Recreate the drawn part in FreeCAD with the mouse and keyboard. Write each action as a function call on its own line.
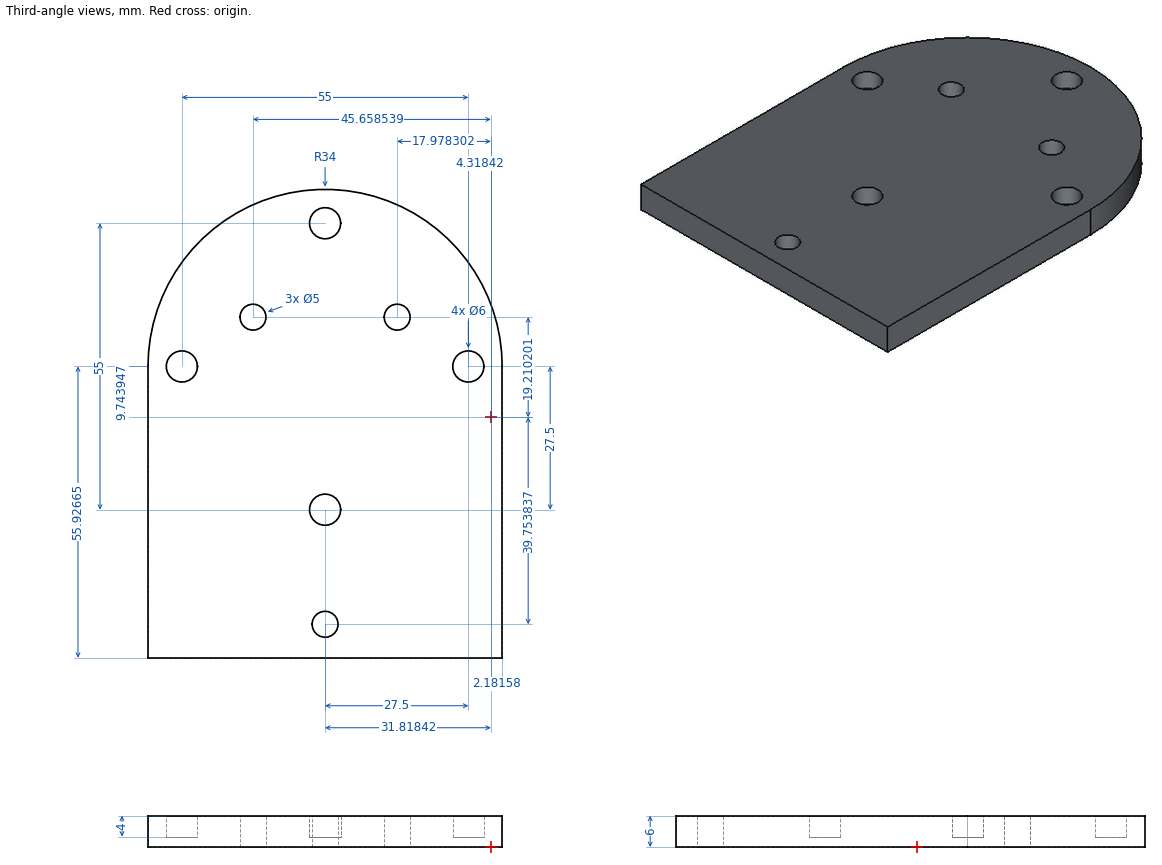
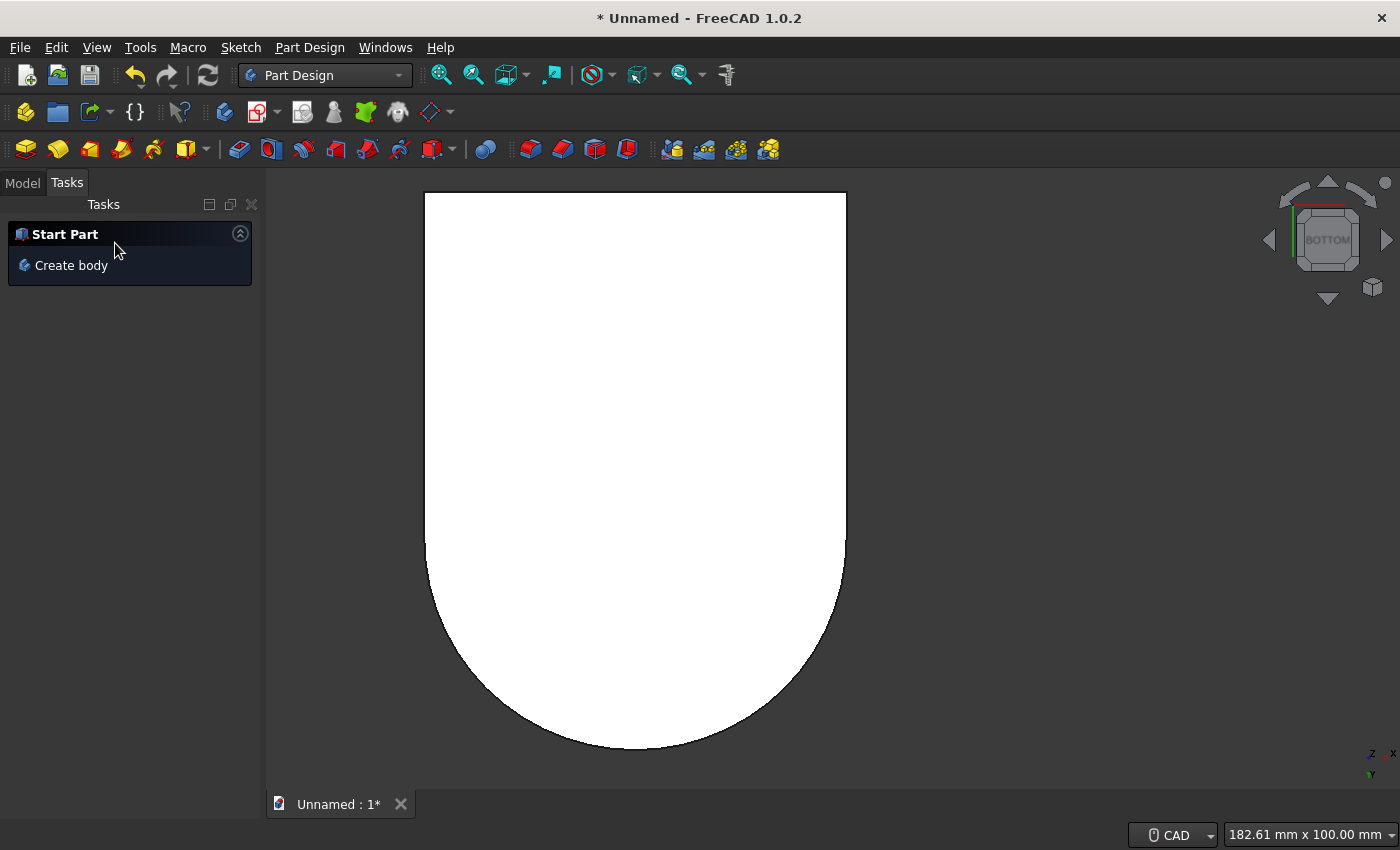
click(635, 470)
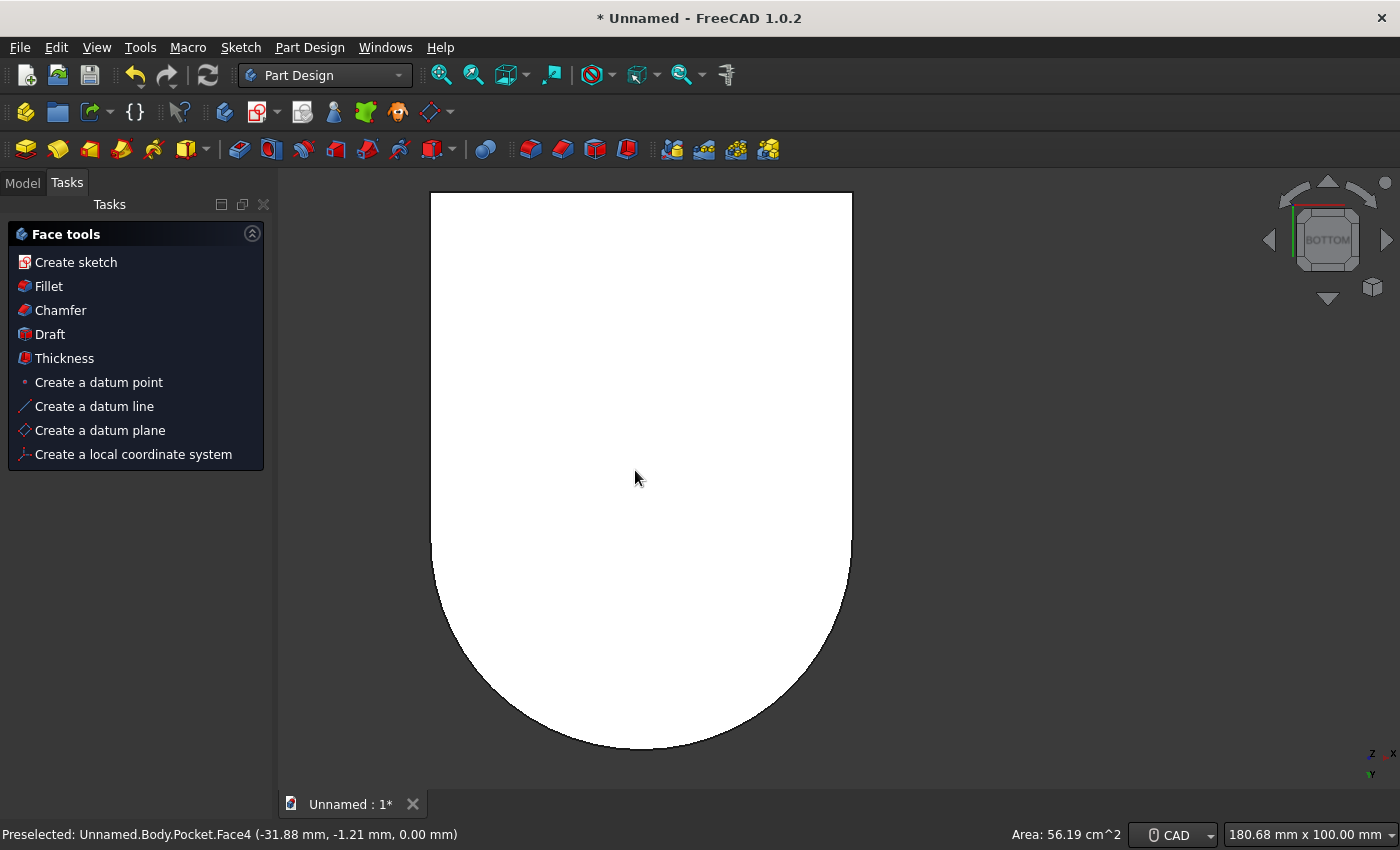
click(258, 112)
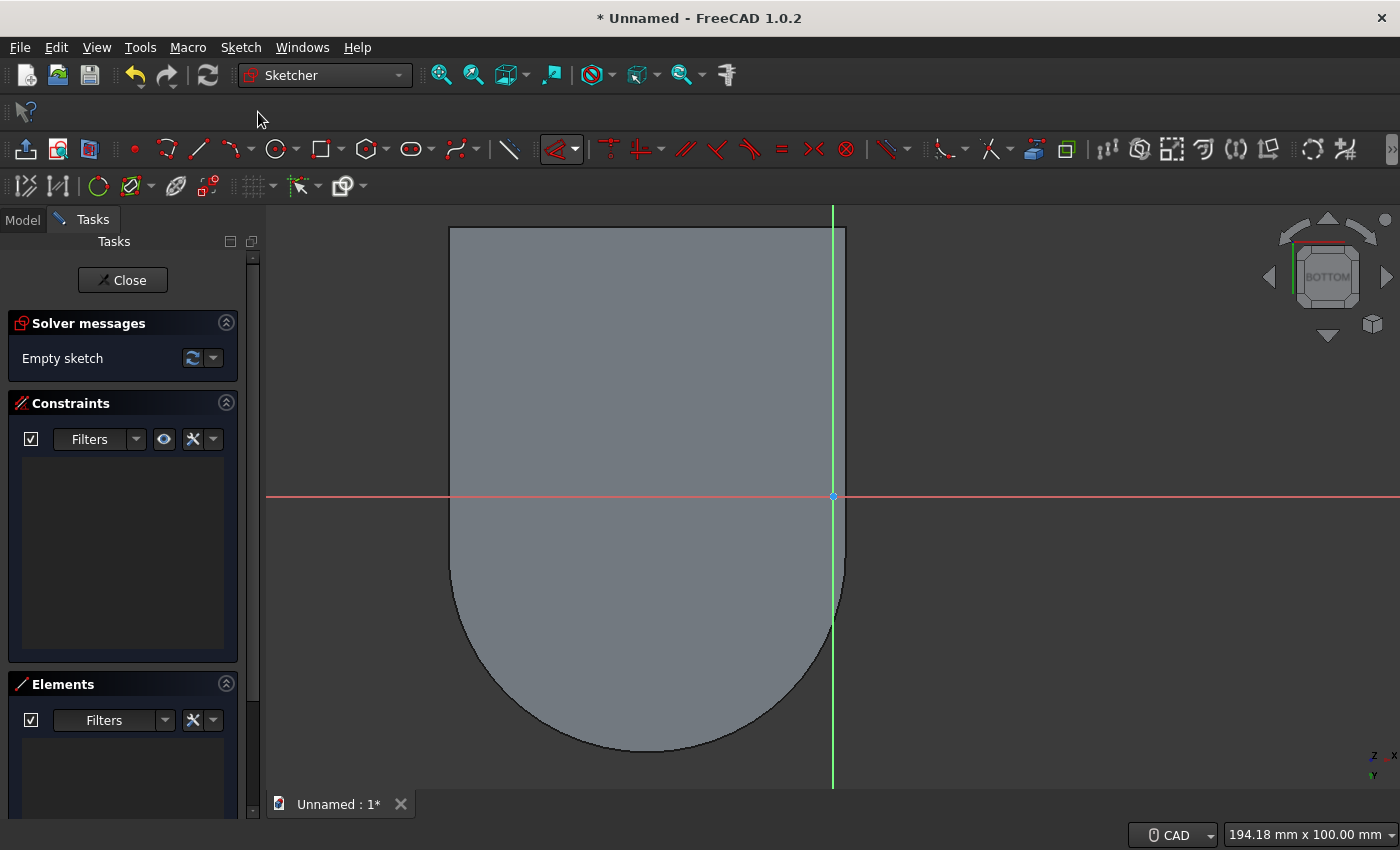
scroll(1090, 761, down, 1)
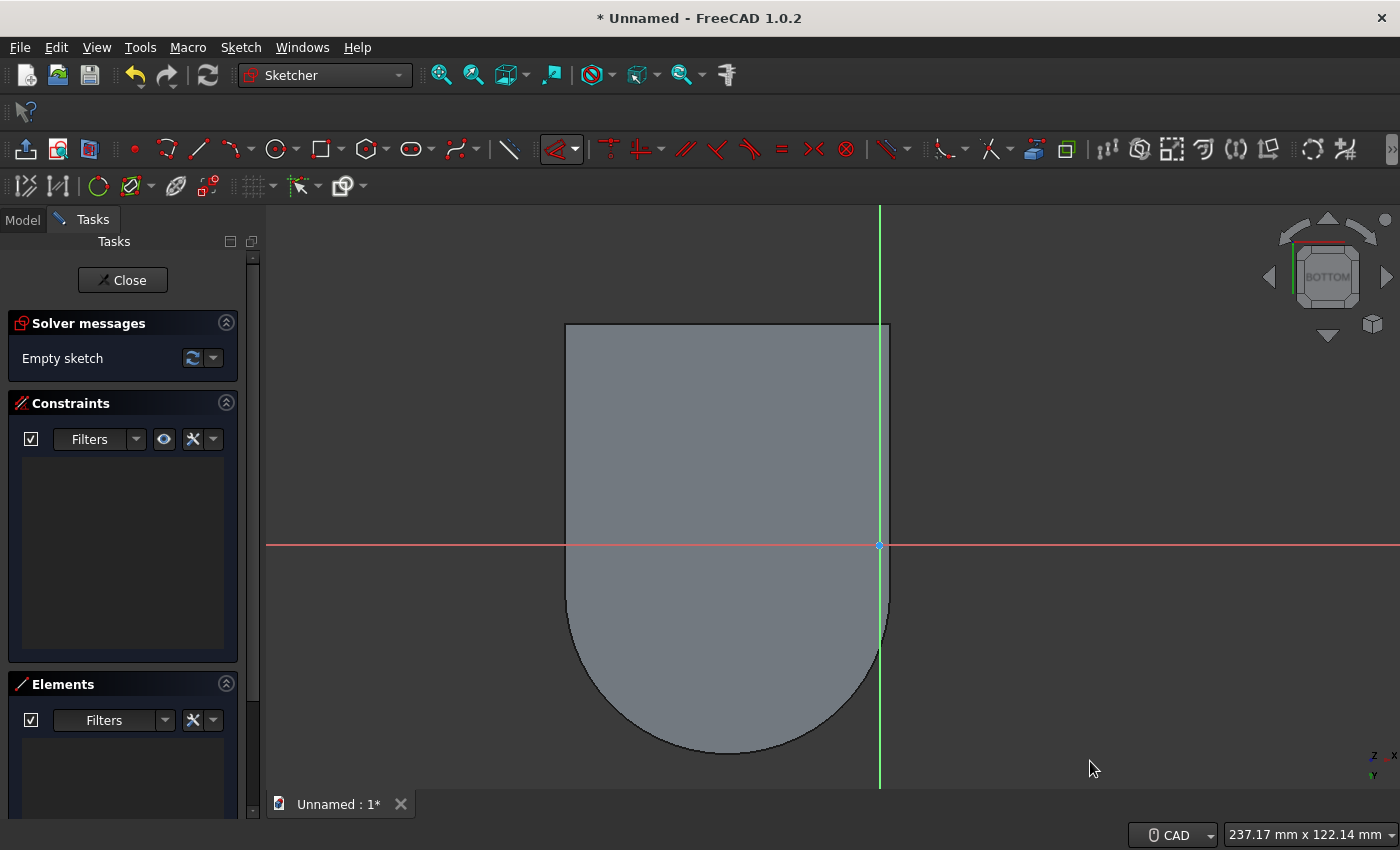
key(g)
key(c)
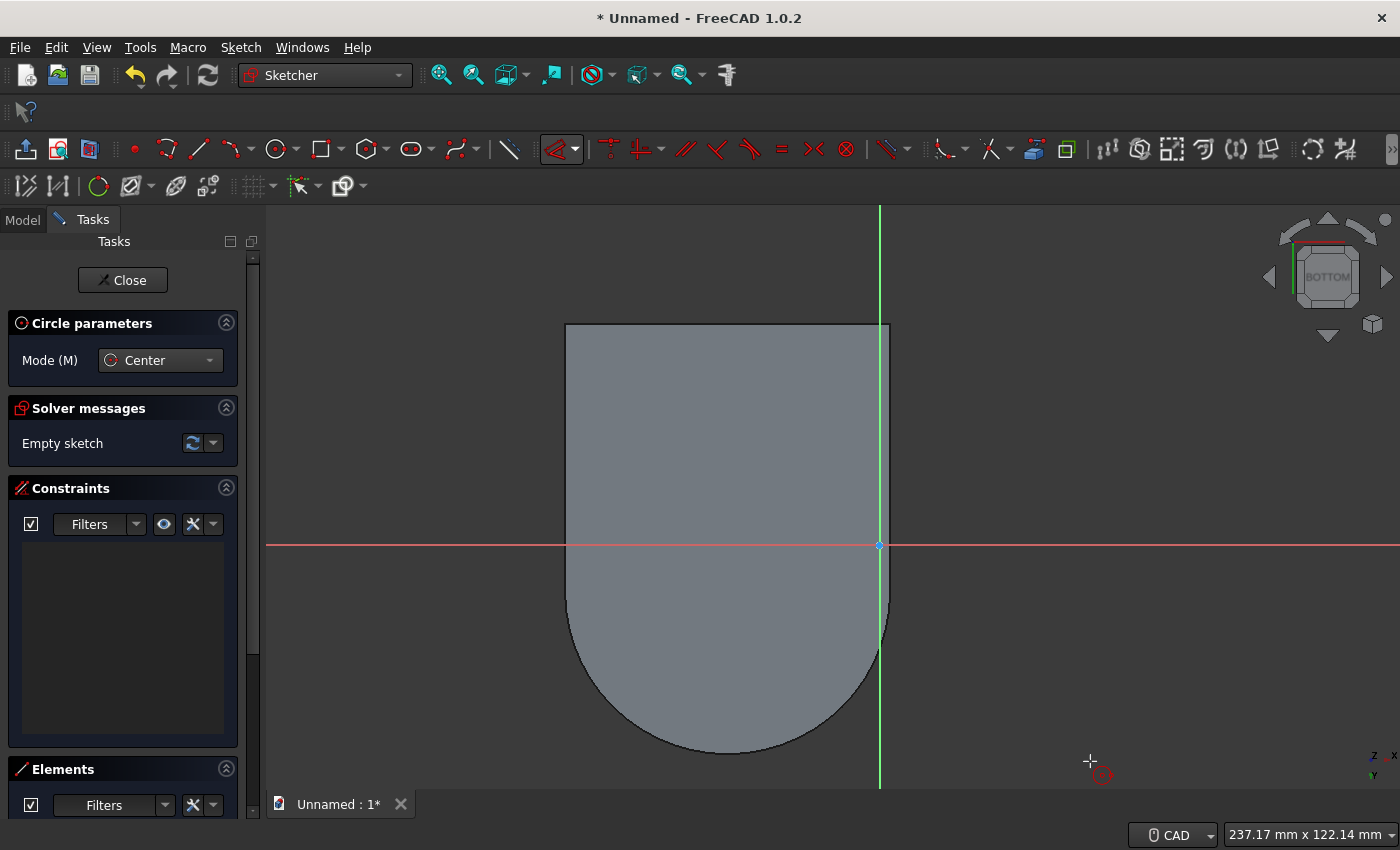
scroll(661, 637, up, 4)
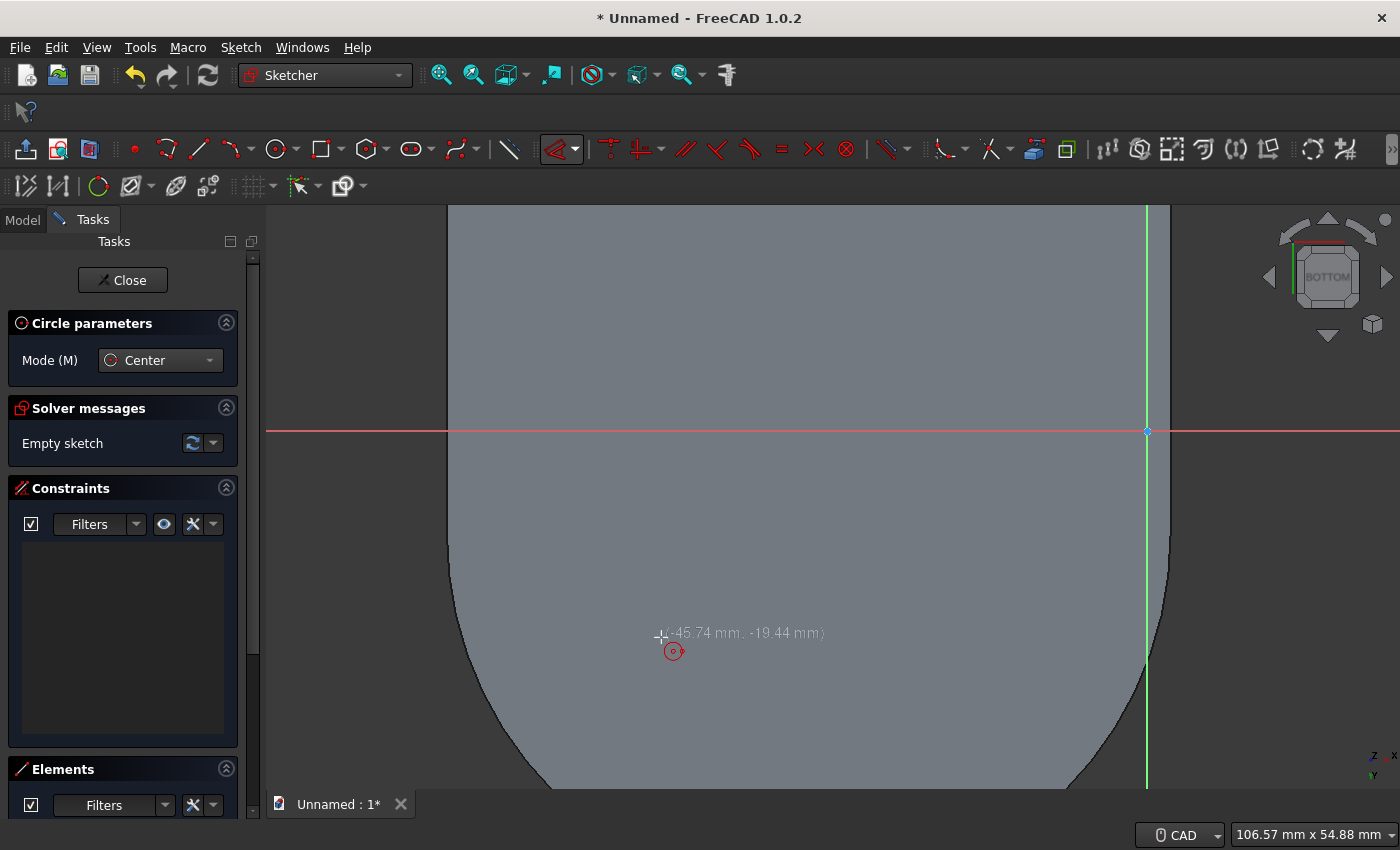
click(661, 636)
click(680, 617)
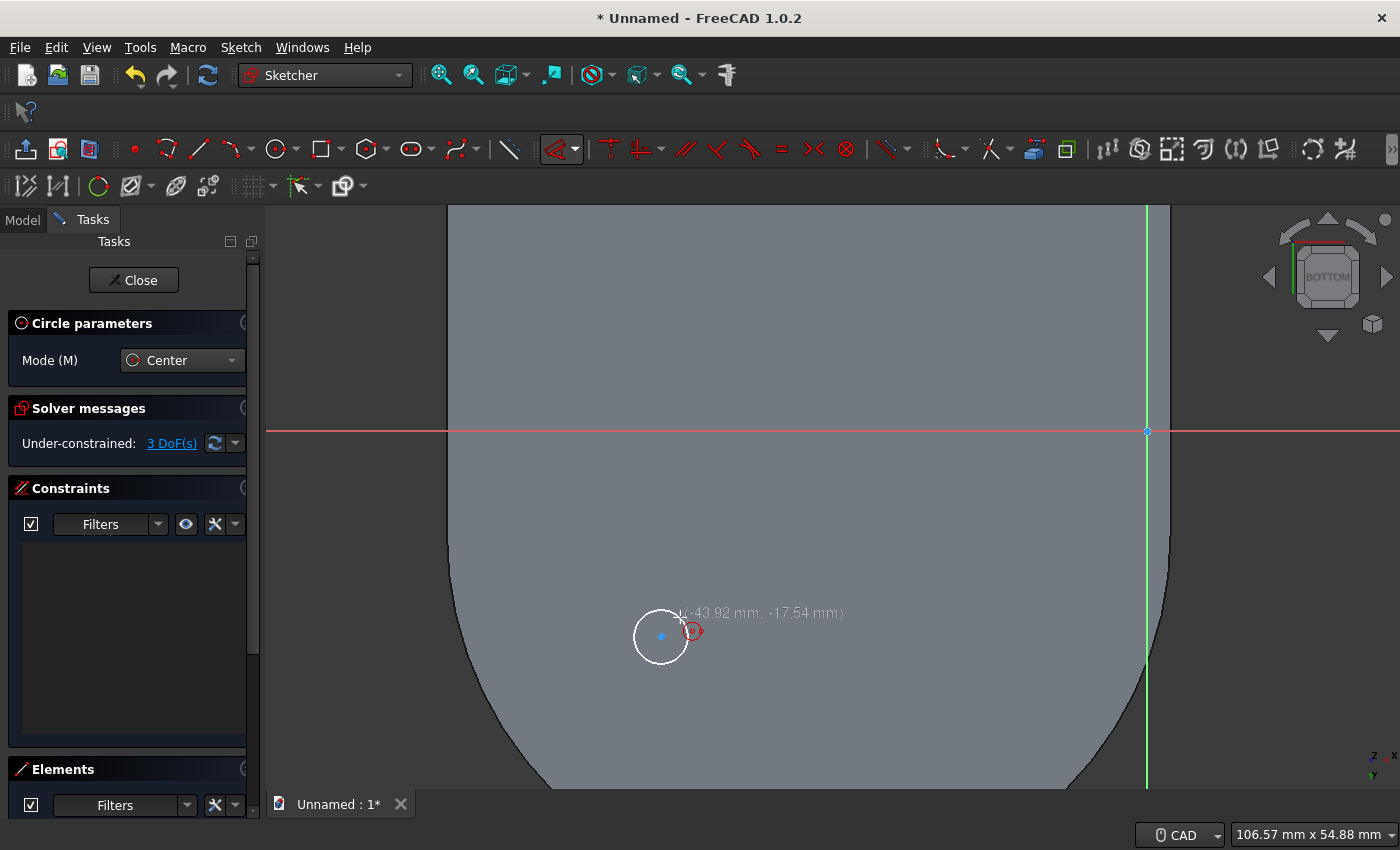
click(956, 636)
click(975, 617)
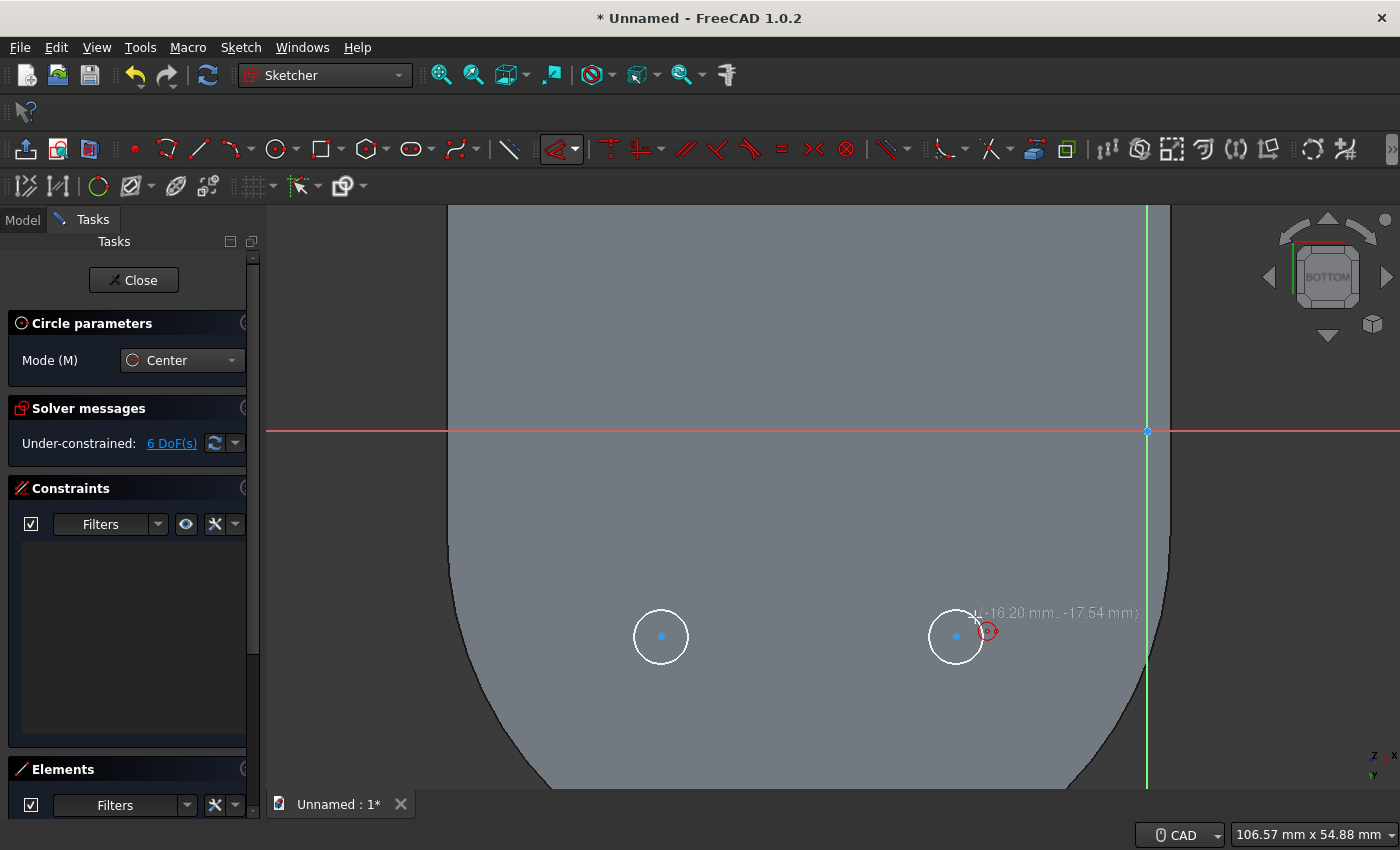
scroll(610, 710, down, 3)